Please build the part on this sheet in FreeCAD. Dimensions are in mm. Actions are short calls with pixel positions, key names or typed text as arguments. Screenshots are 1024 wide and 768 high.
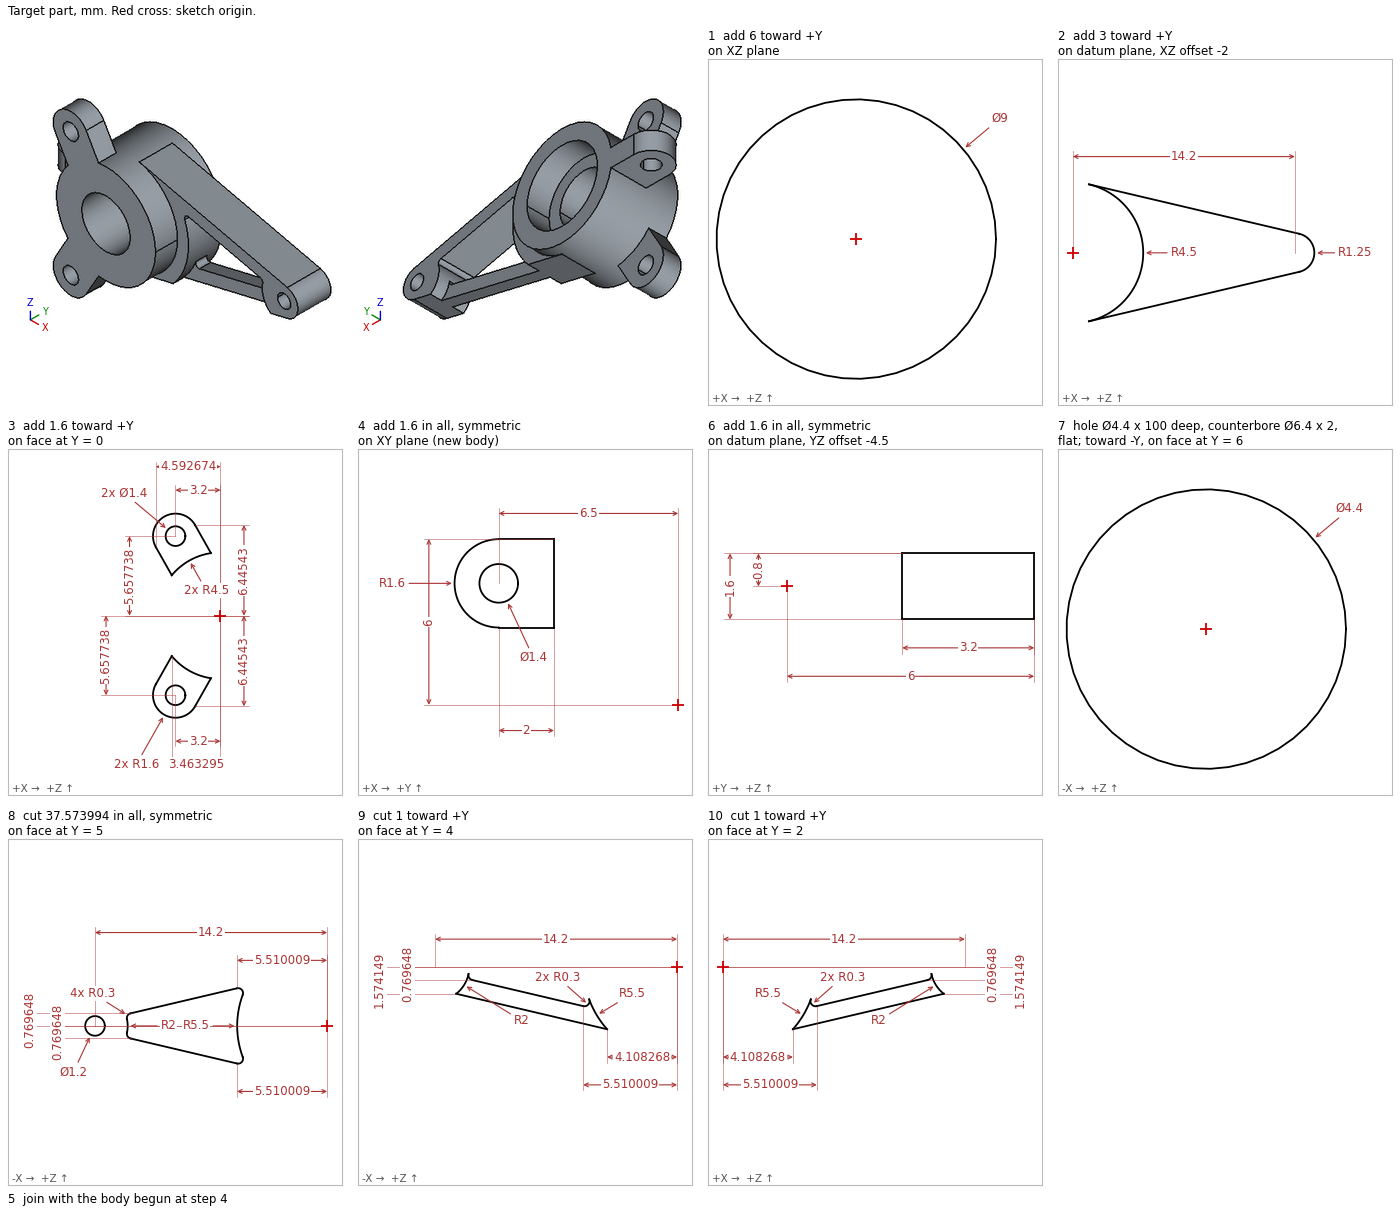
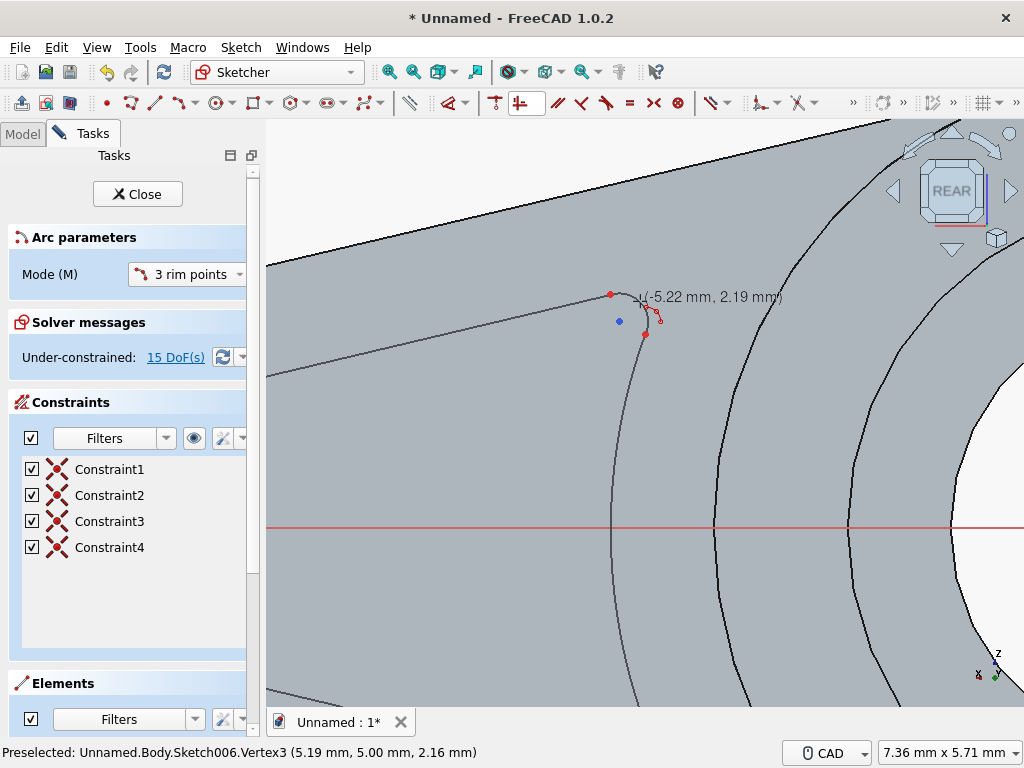
scroll(629, 375, down, 7)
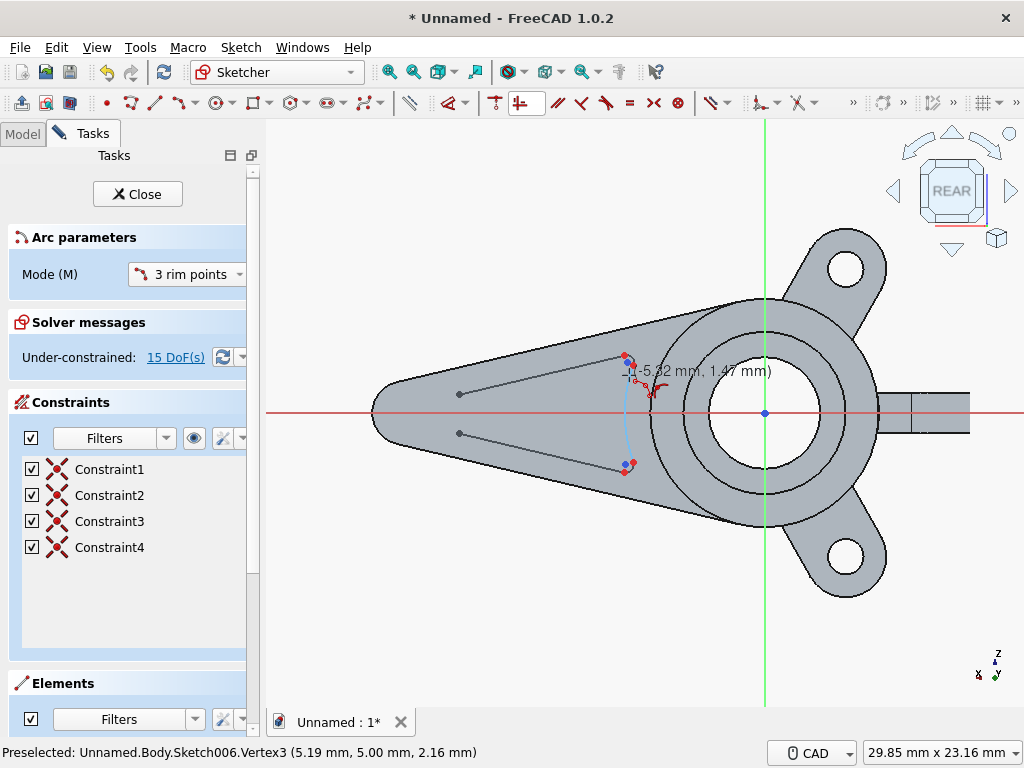
click(460, 395)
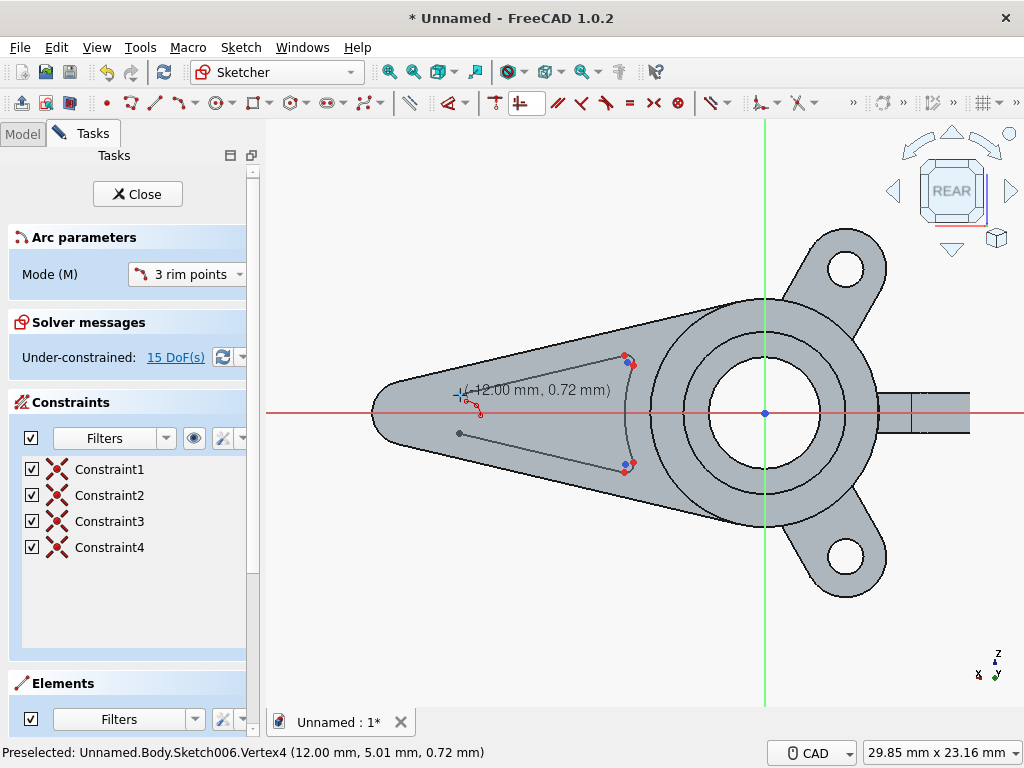
scroll(454, 402, up, 3)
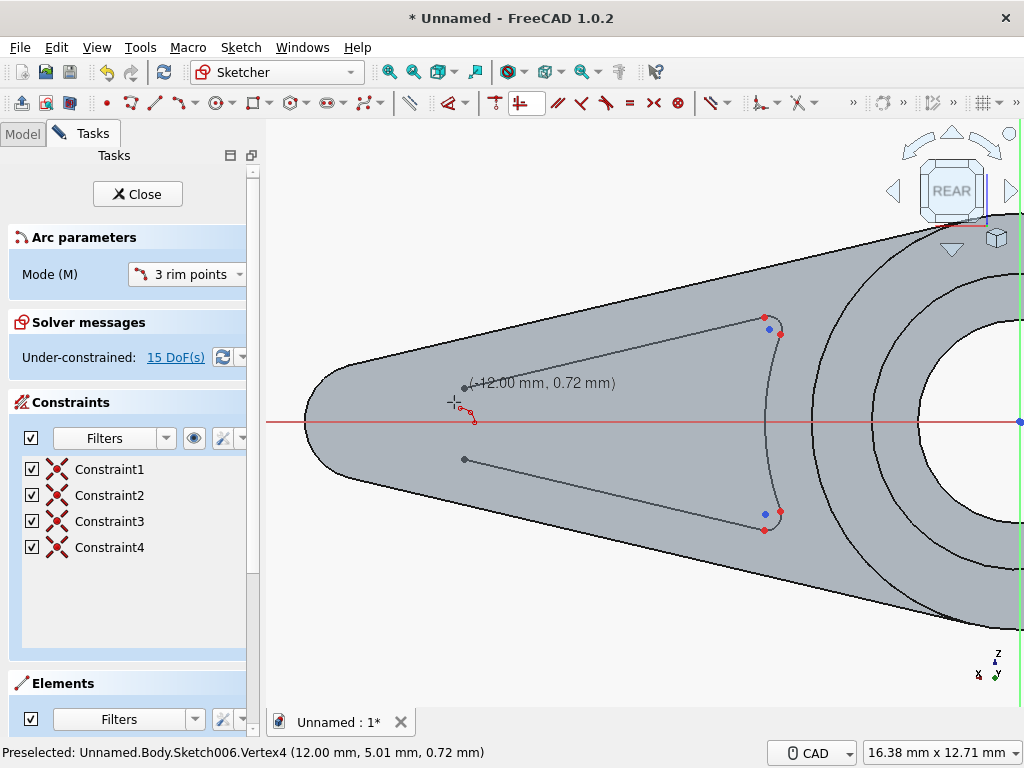
click(453, 402)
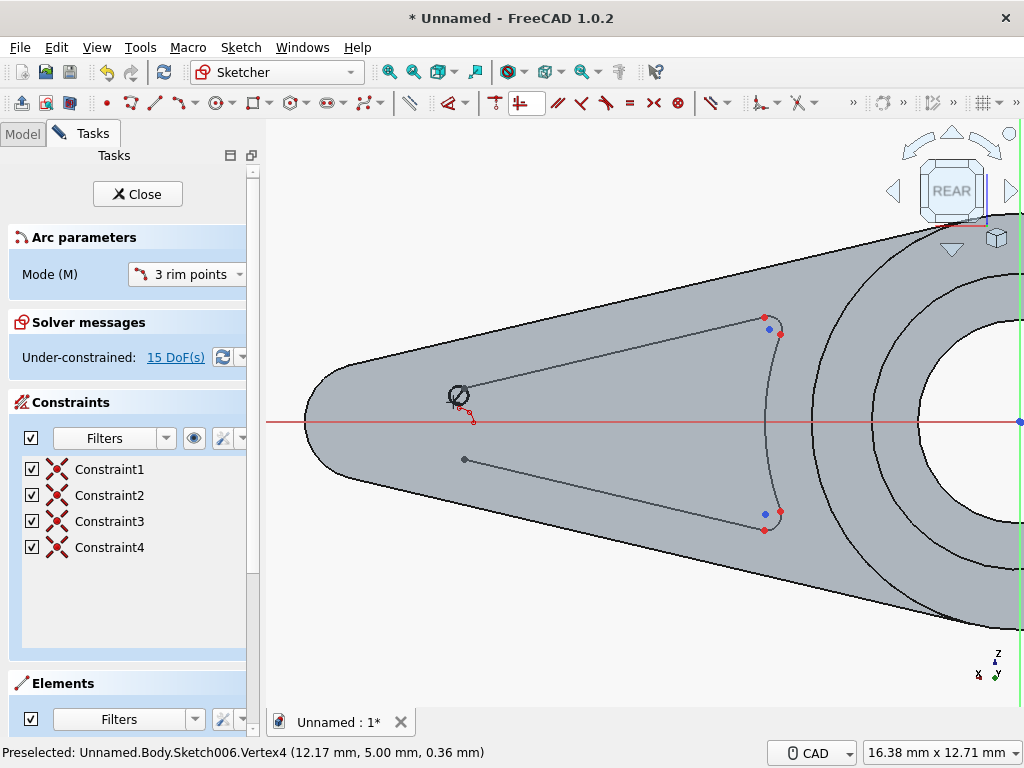
scroll(455, 392, up, 7)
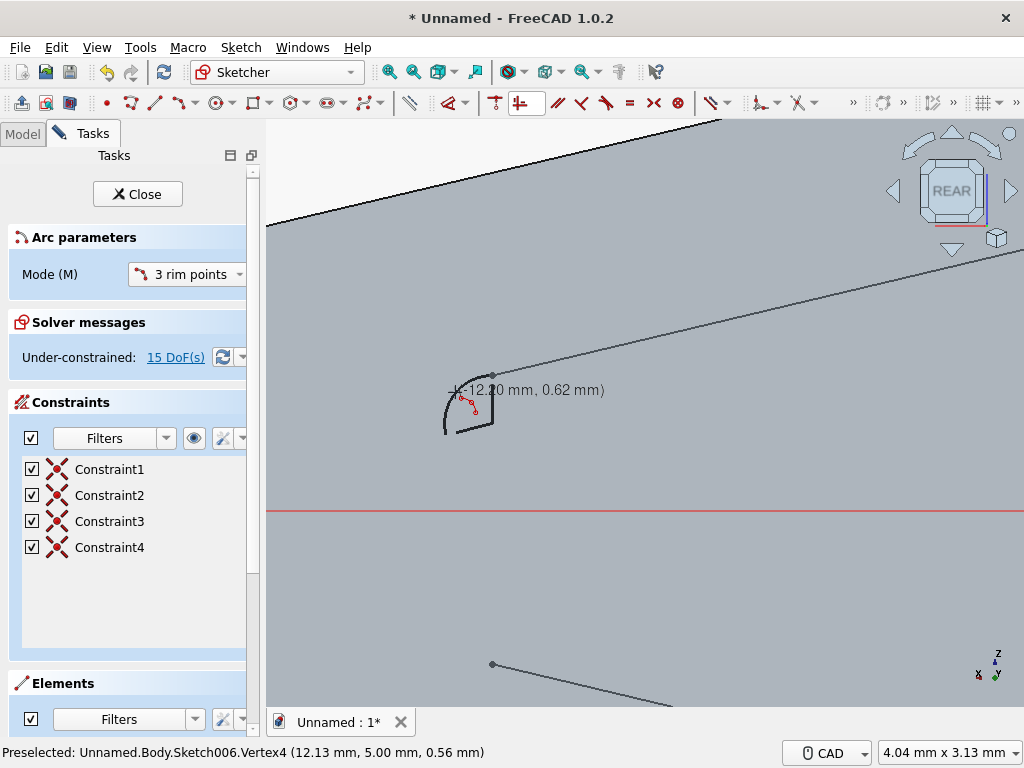
click(454, 391)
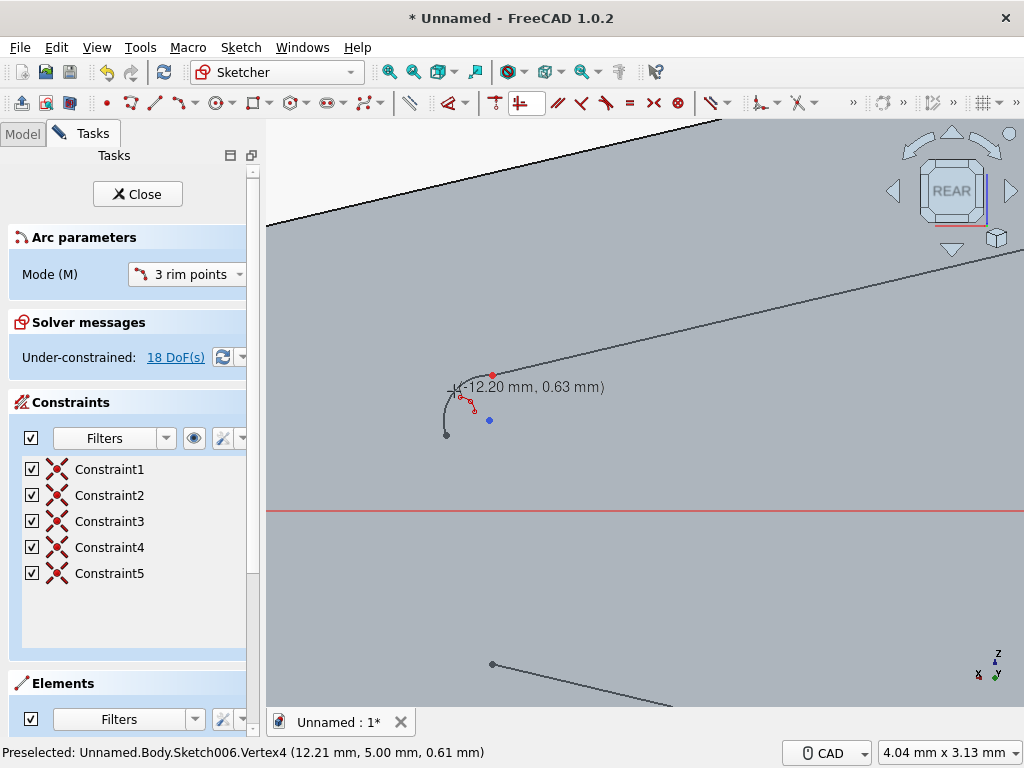
scroll(455, 398, down, 10)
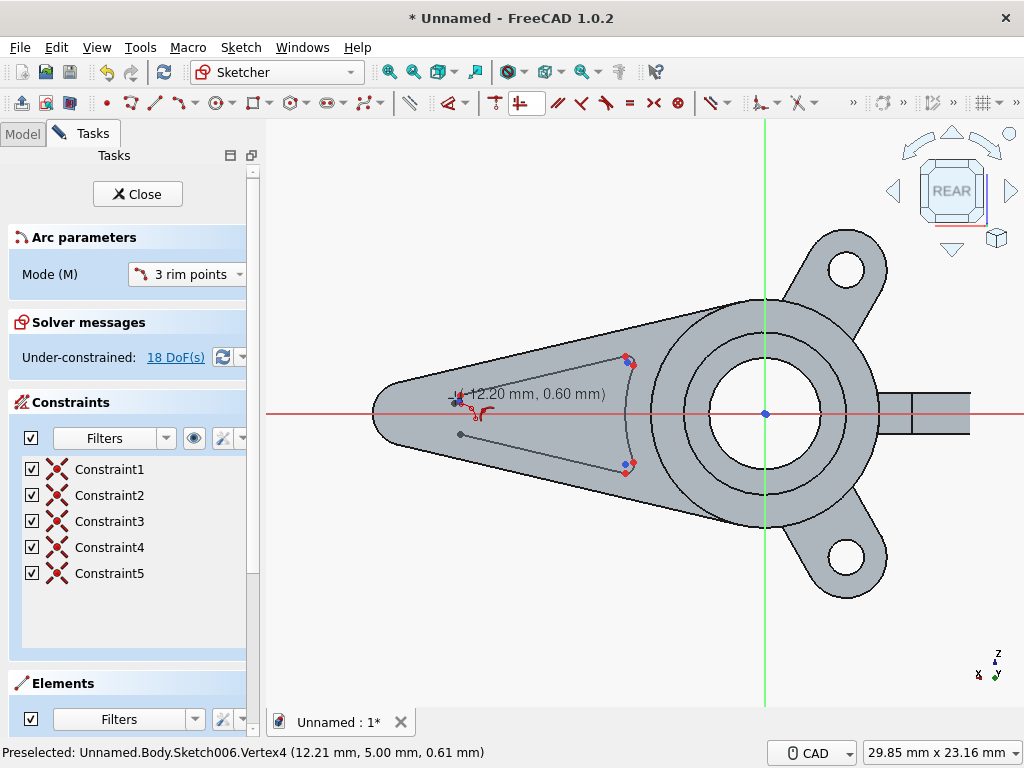
scroll(454, 403, up, 4)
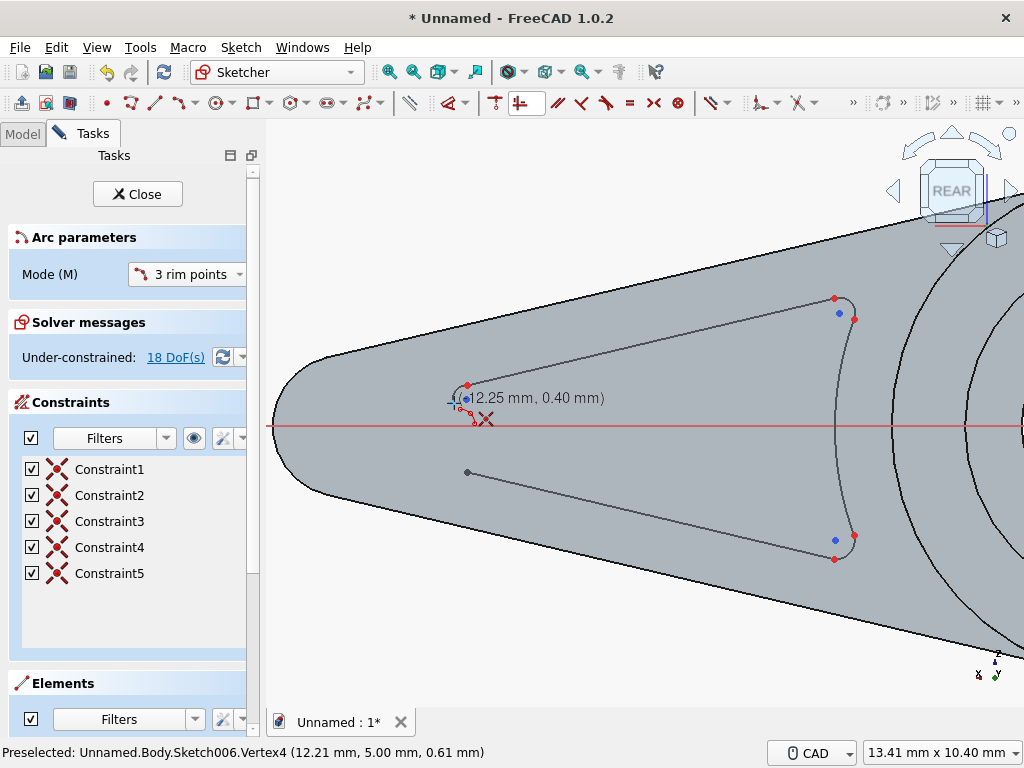
click(454, 403)
click(454, 450)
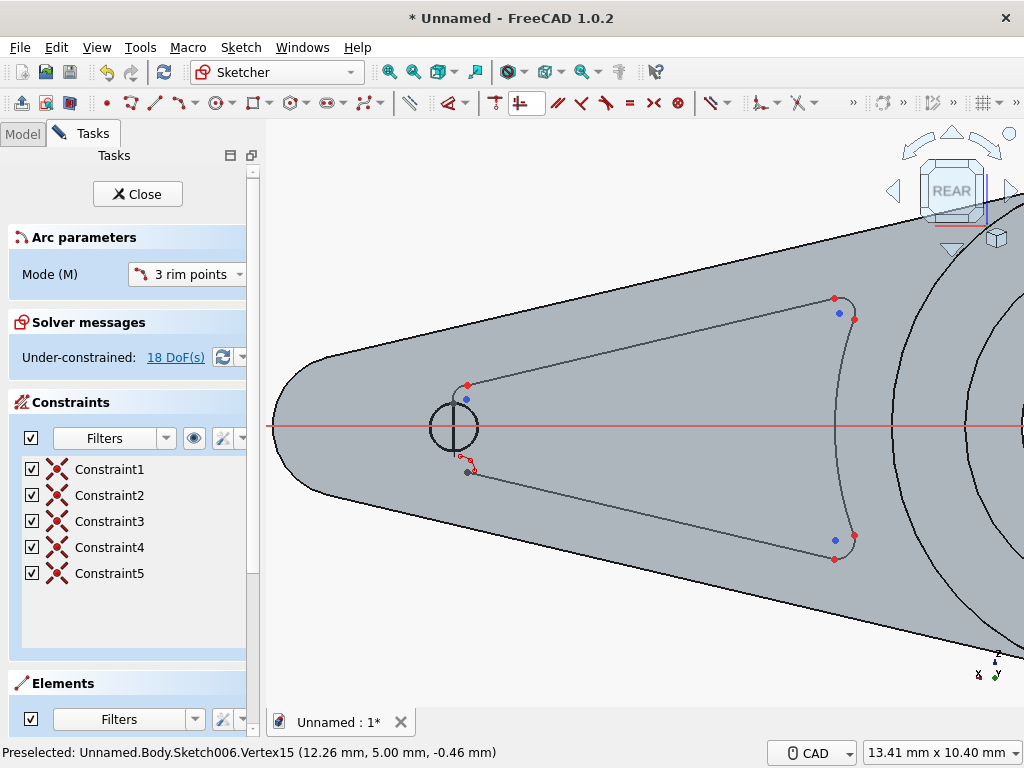
scroll(456, 431, up, 10)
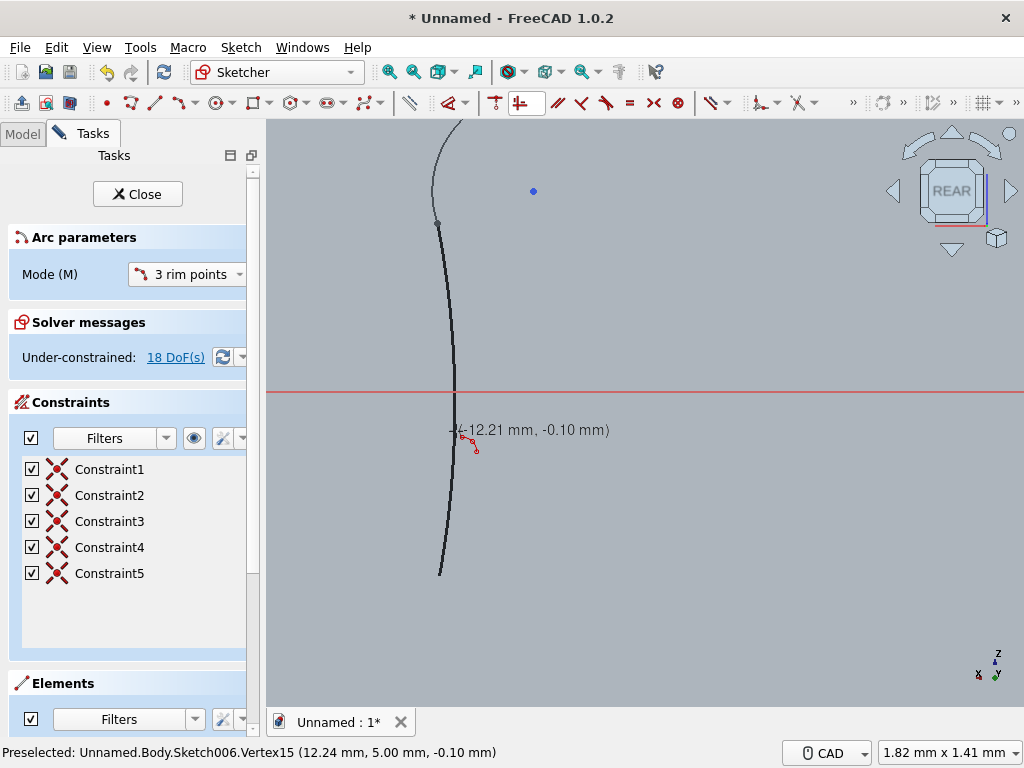
click(456, 427)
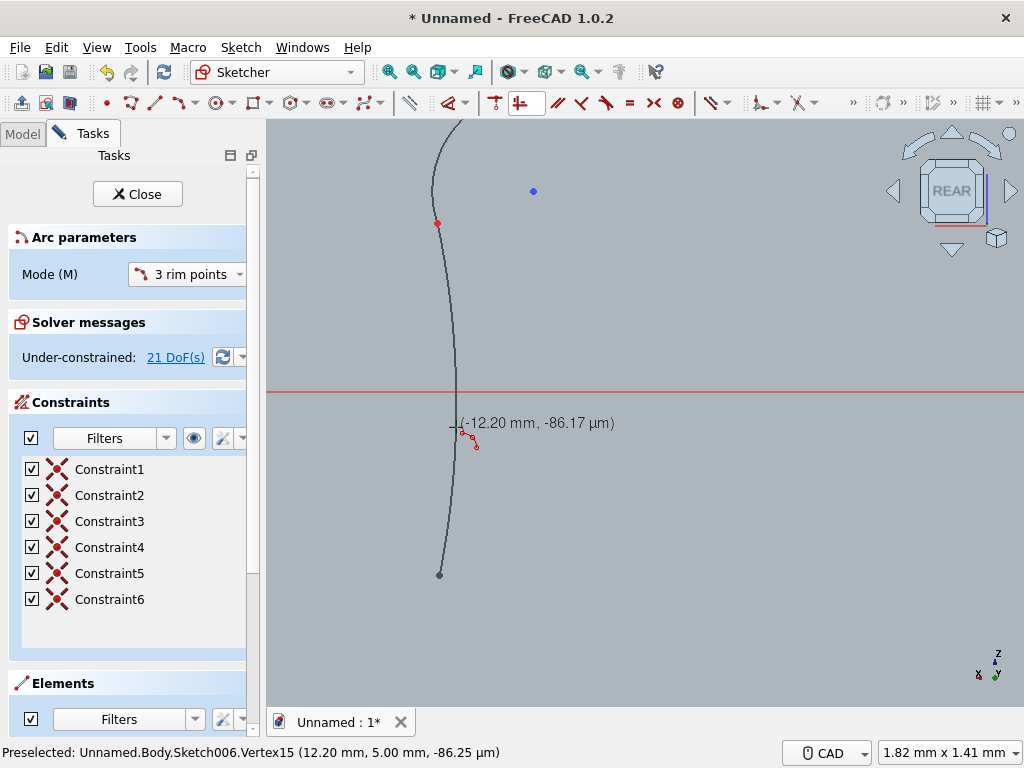
scroll(454, 414, down, 14)